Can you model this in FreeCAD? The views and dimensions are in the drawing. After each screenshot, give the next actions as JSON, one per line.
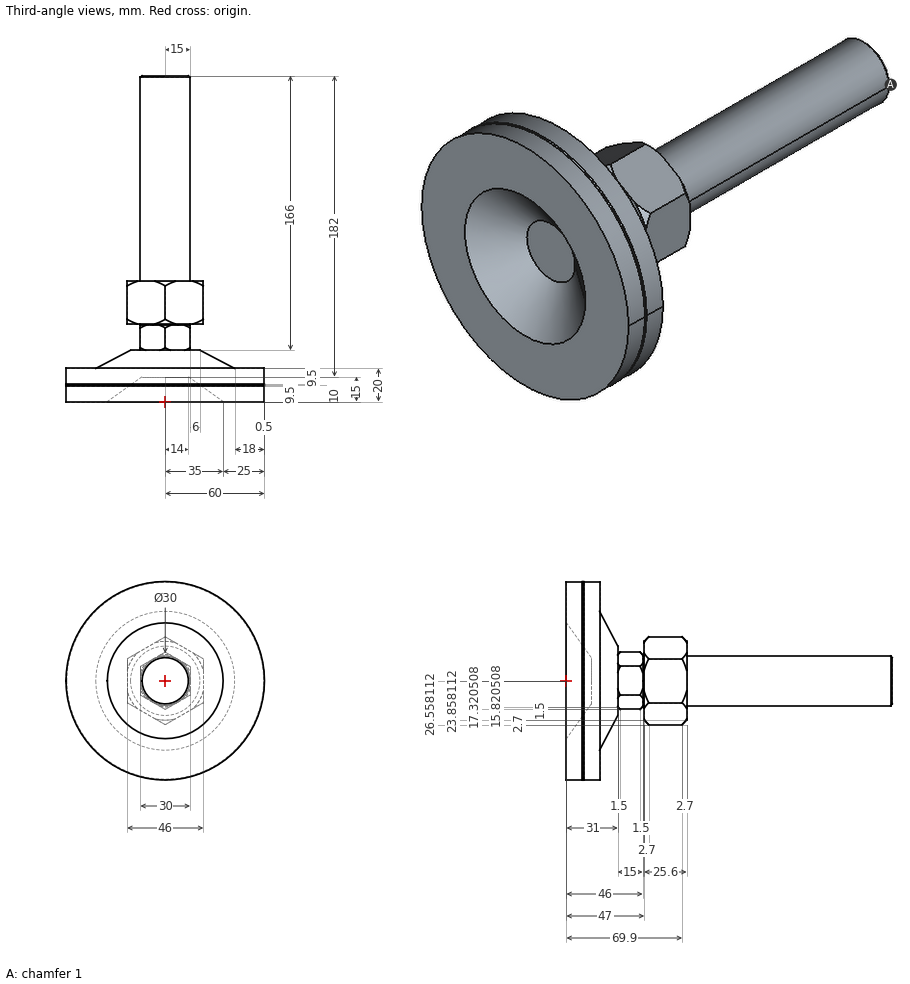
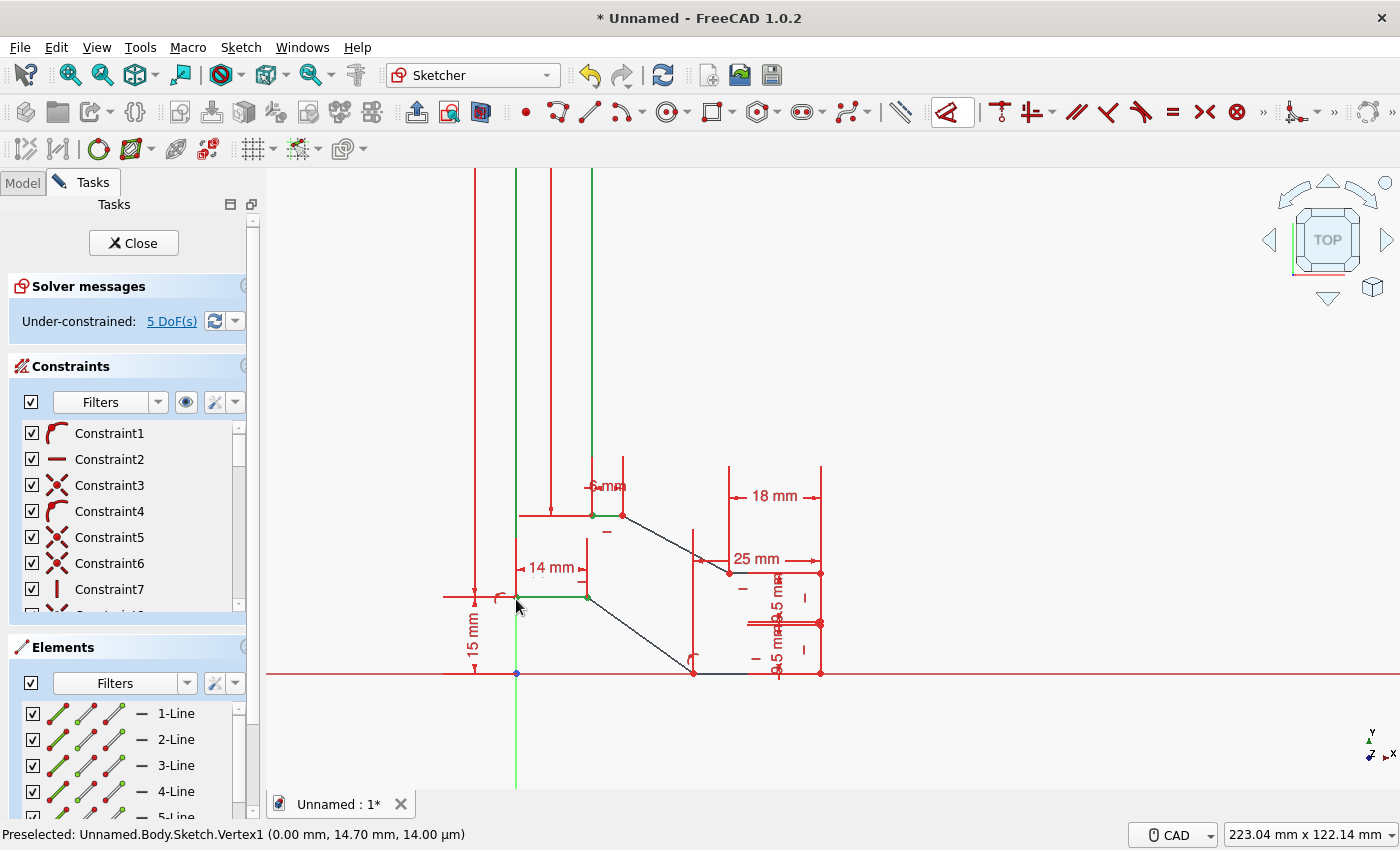
{"action": "left_click", "coordinate": [693, 674]}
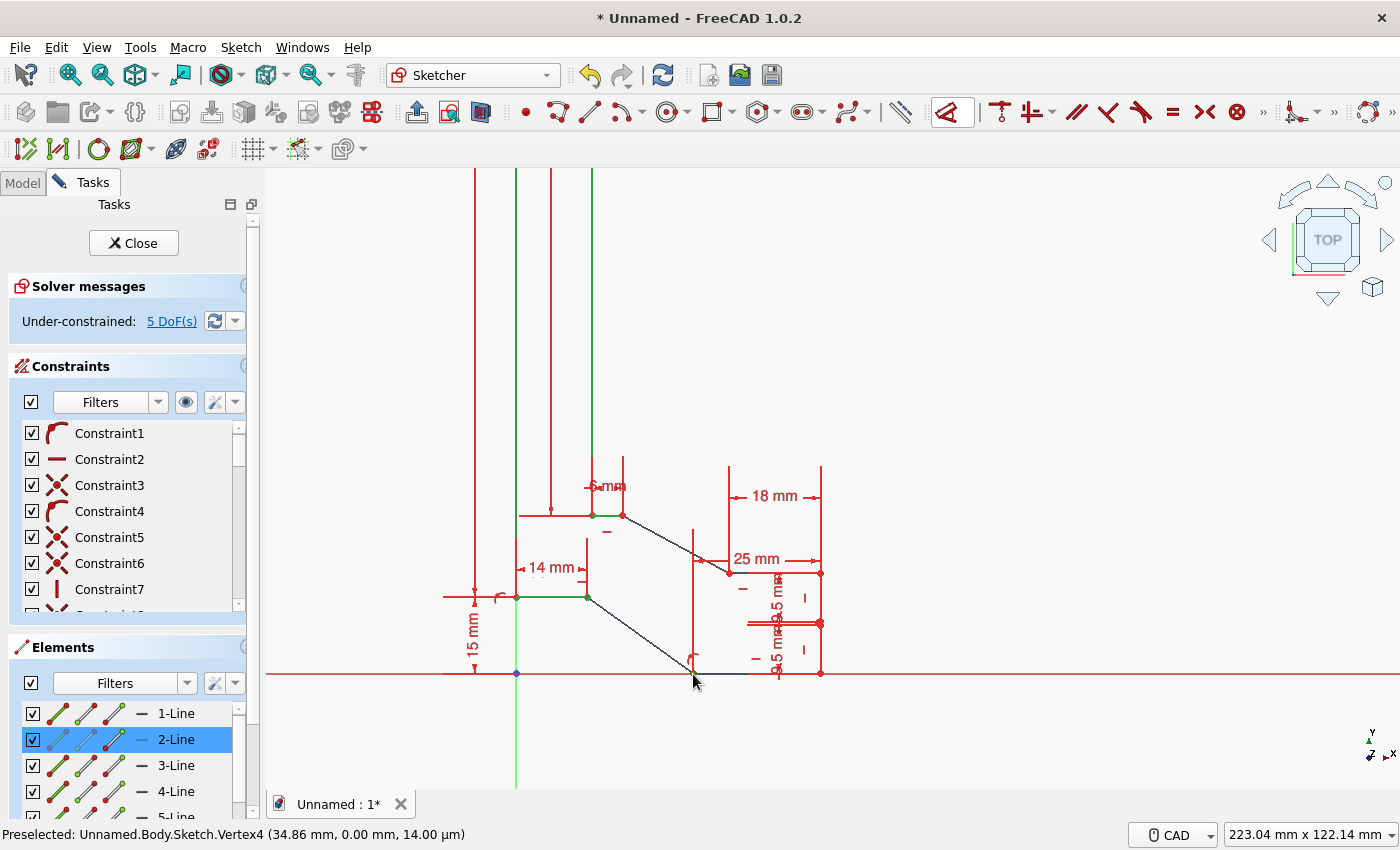
{"action": "left_click", "coordinate": [968, 112]}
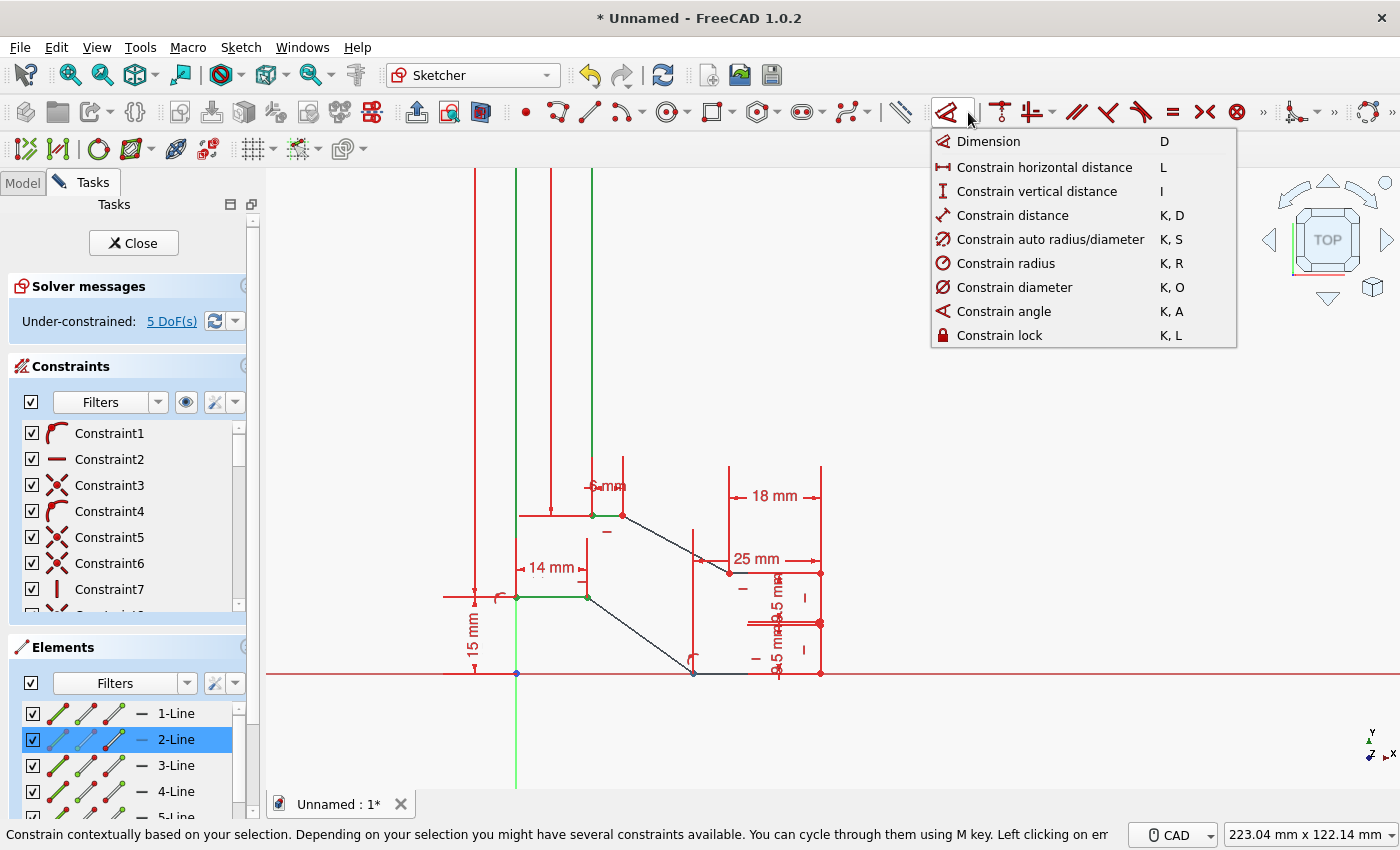
{"action": "left_click", "coordinate": [1084, 167]}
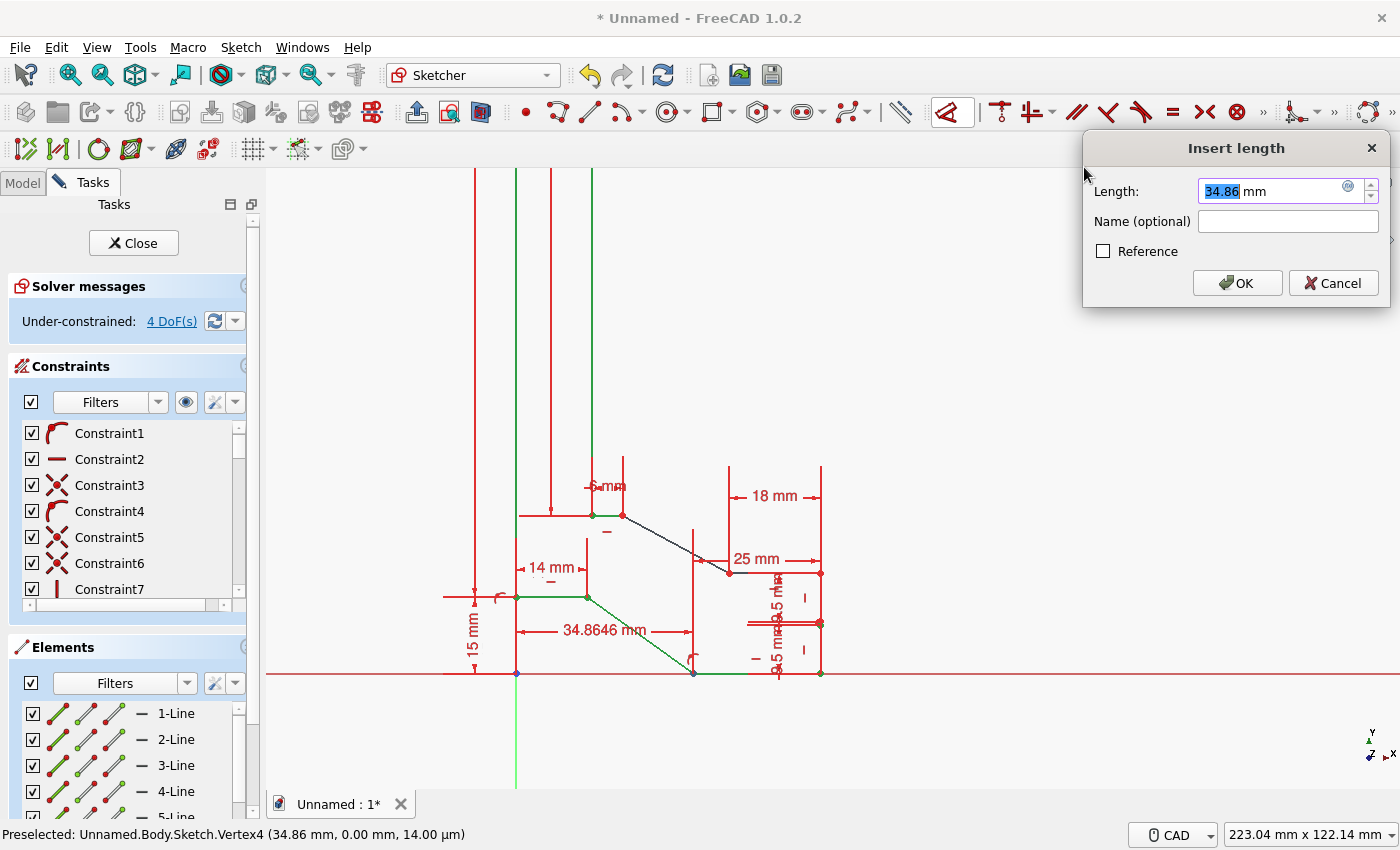
{"action": "type", "text": "35"}
{"action": "key", "text": "Return"}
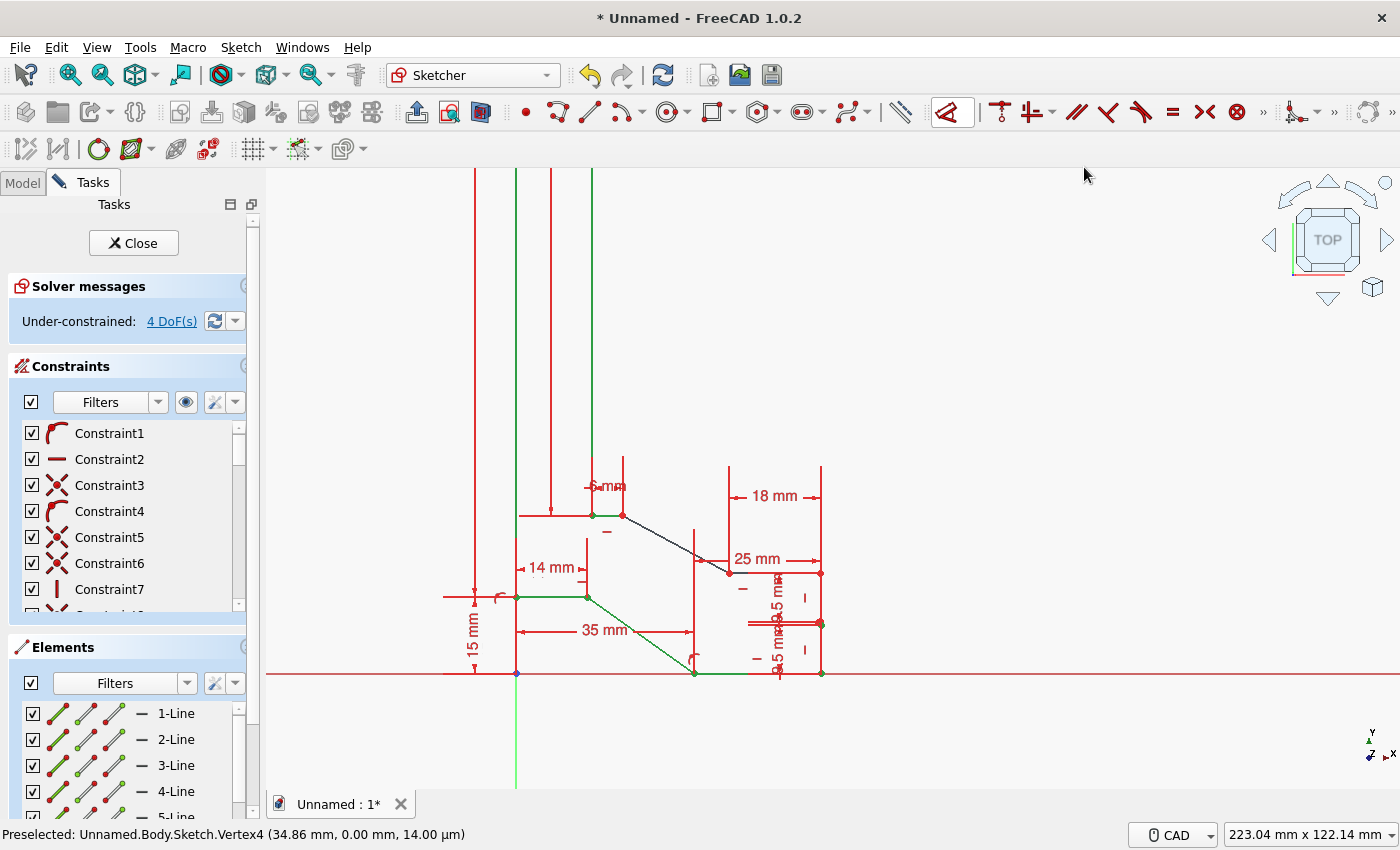
{"action": "scroll", "coordinate": [819, 623], "scroll_direction": "up", "scroll_amount": 9}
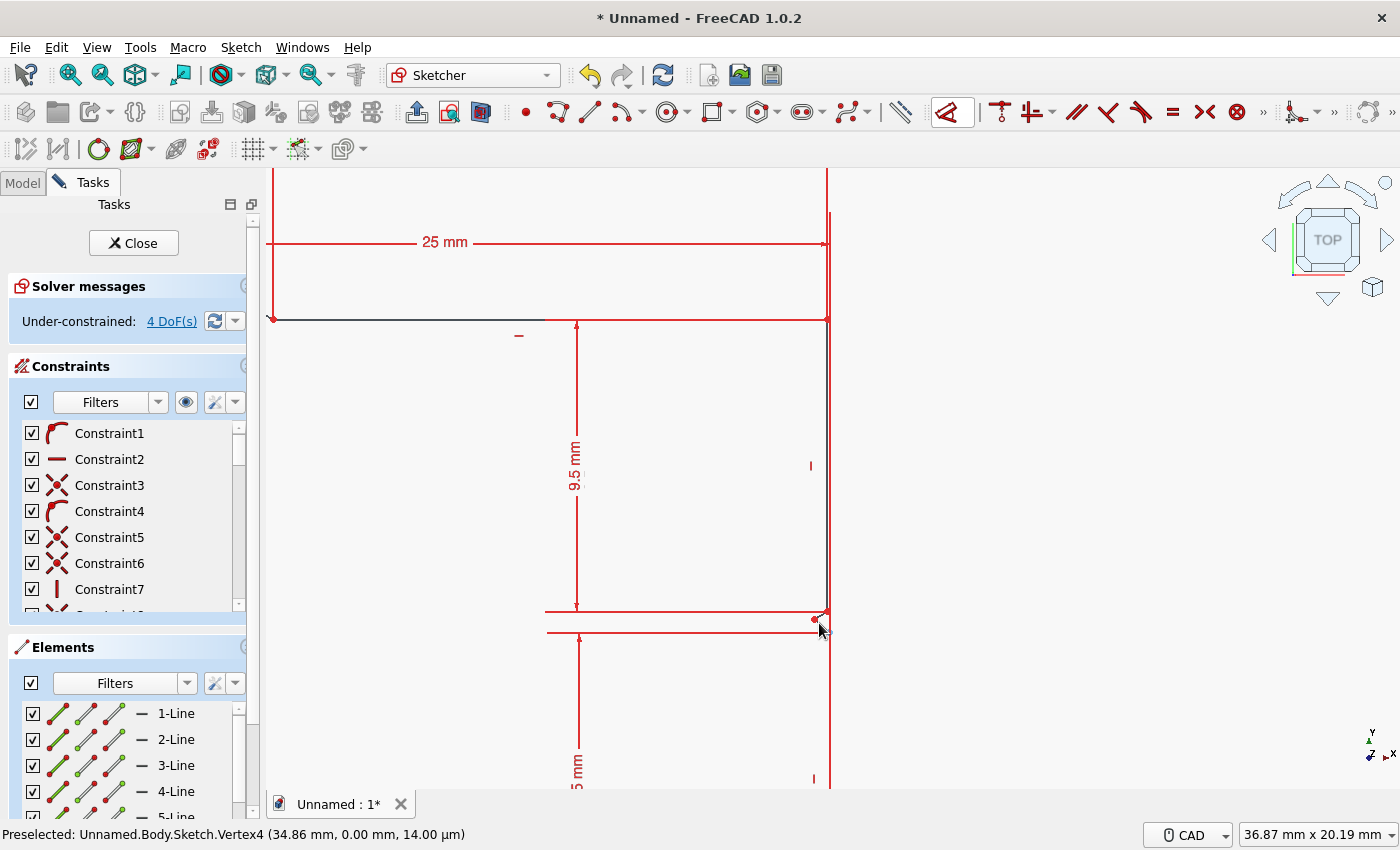
{"action": "left_click", "coordinate": [815, 619]}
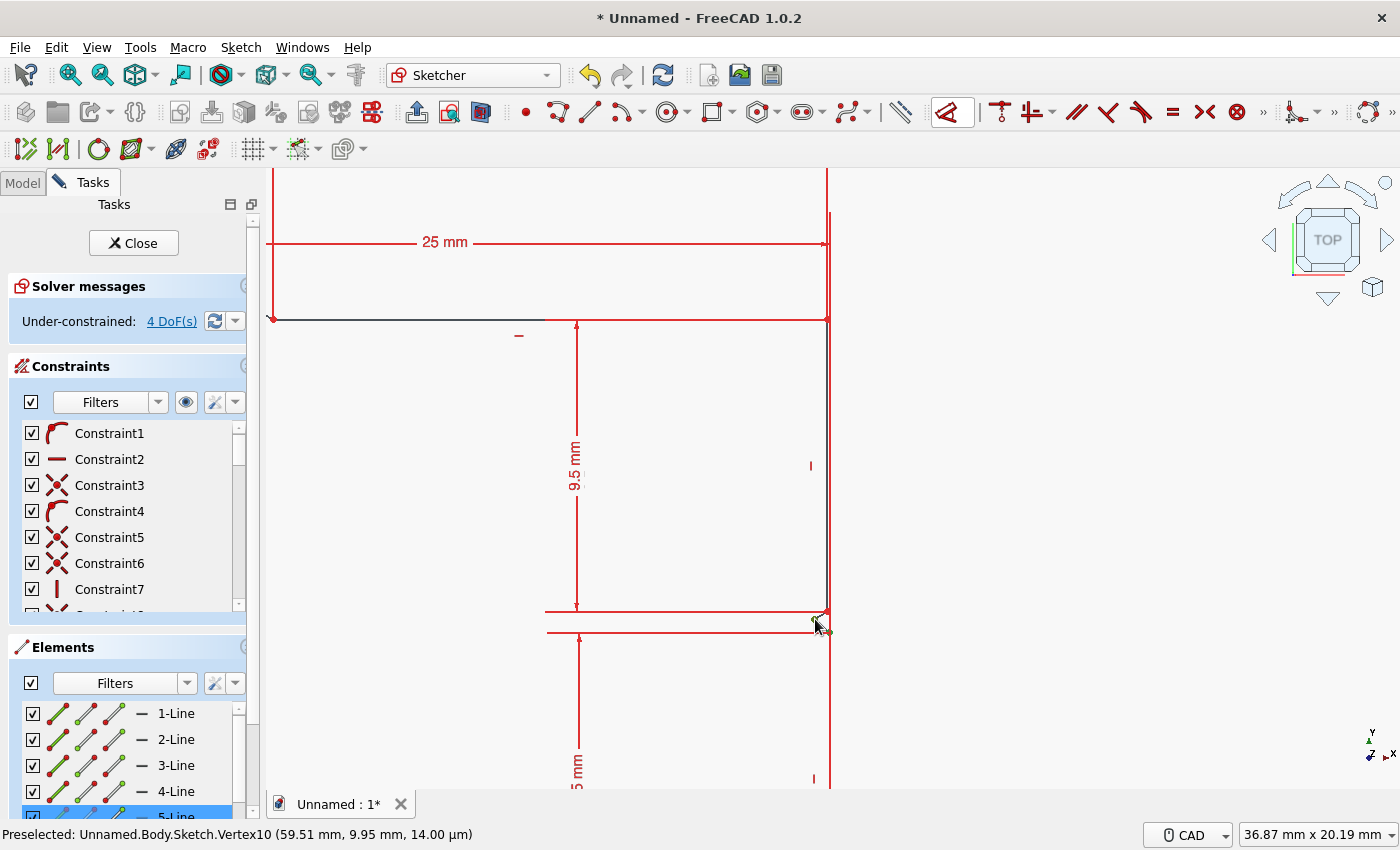
{"action": "key", "text": "i"}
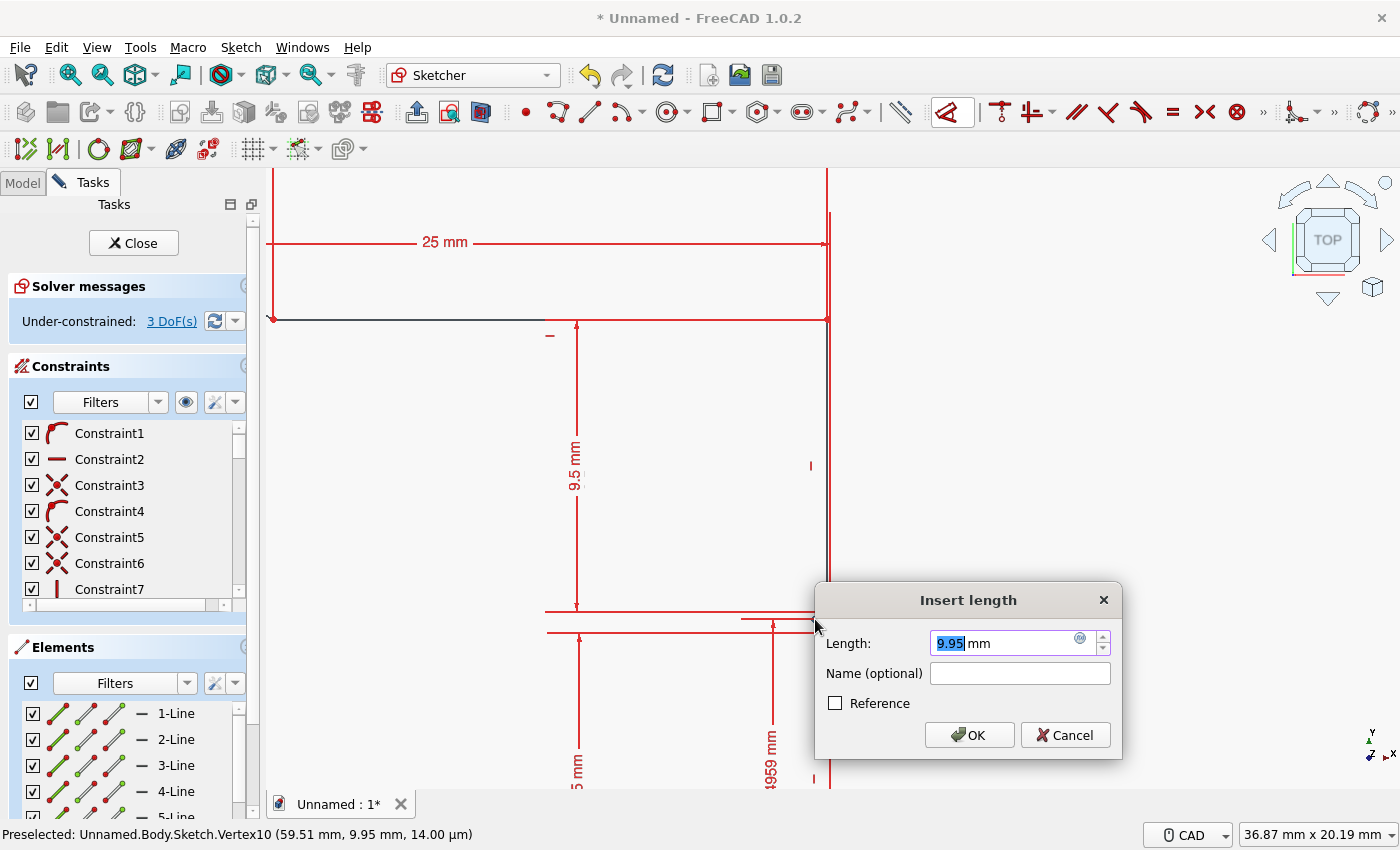
{"action": "type", "text": "10"}
{"action": "key", "text": "Return"}